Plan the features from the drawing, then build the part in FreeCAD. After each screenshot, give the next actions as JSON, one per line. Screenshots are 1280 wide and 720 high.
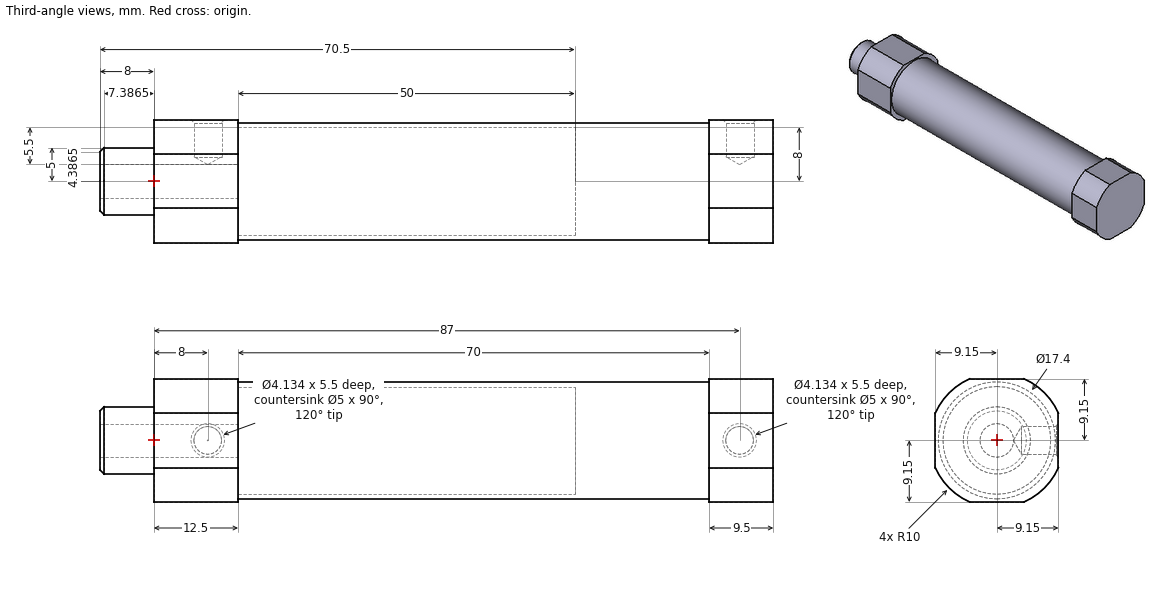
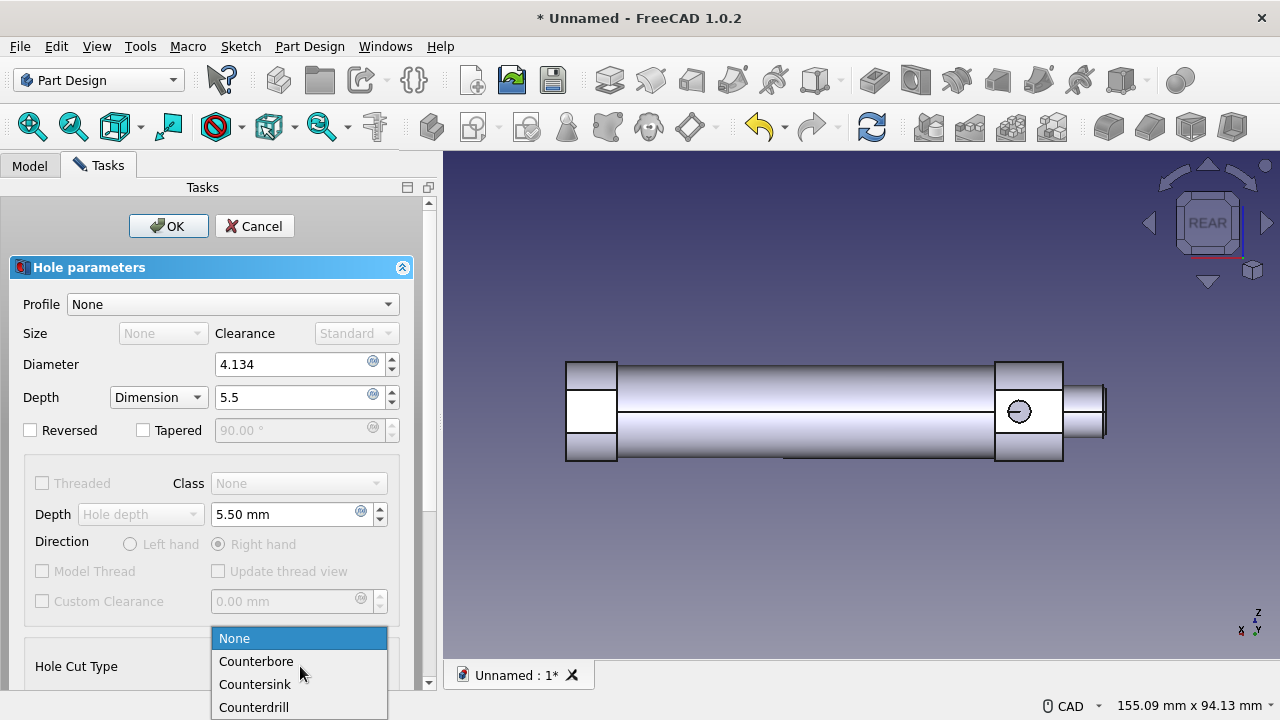
{"action": "left_click", "coordinate": [298, 684]}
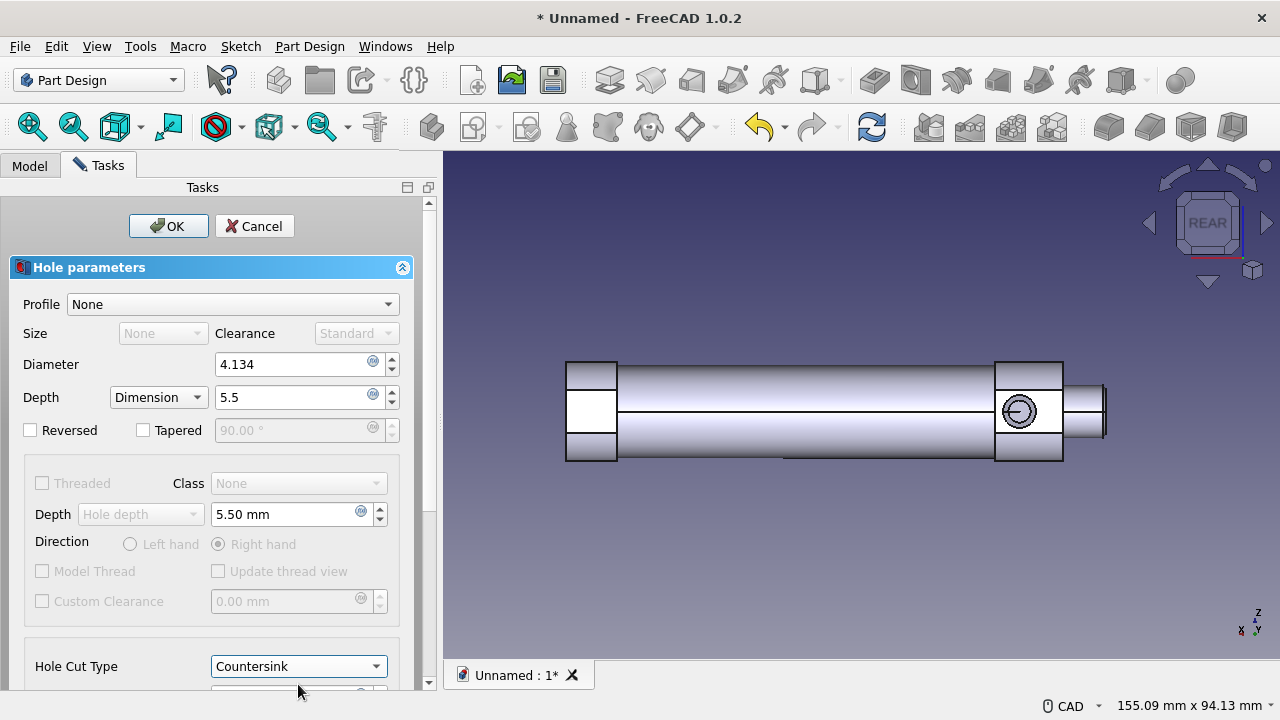
{"action": "scroll", "coordinate": [429, 444], "scroll_direction": "down", "scroll_amount": 2}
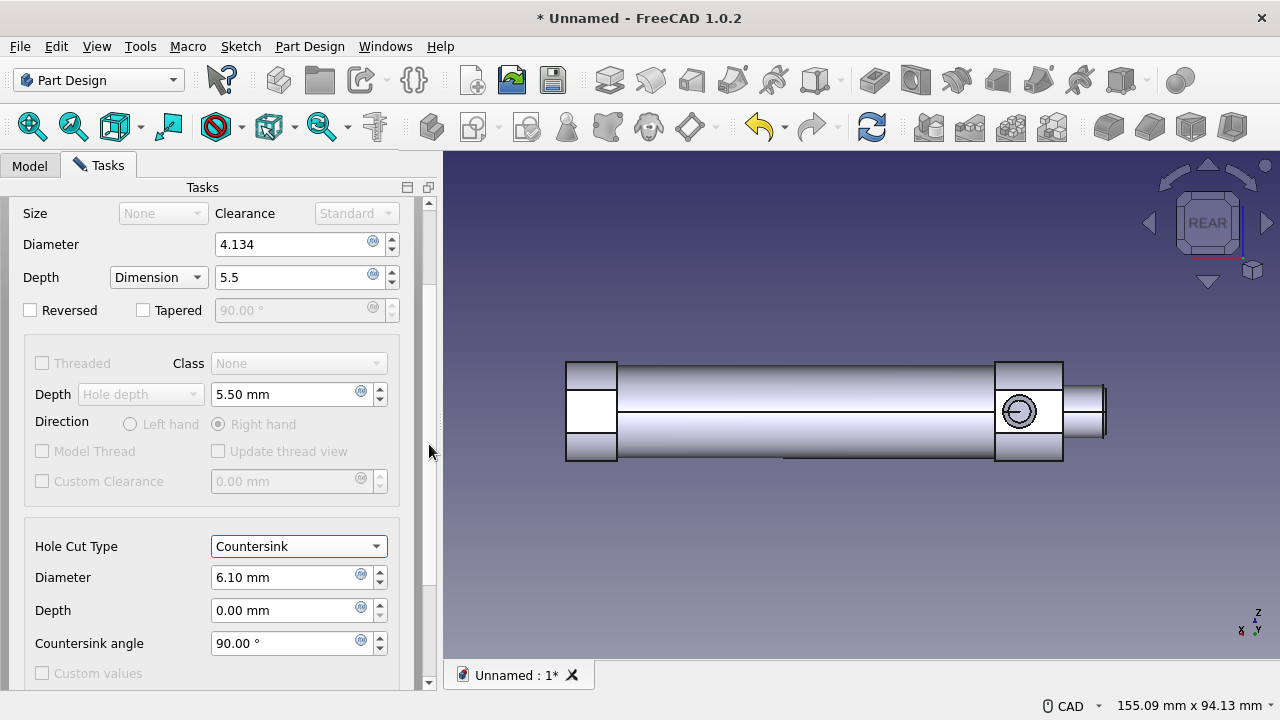
{"action": "triple_click", "coordinate": [292, 578]}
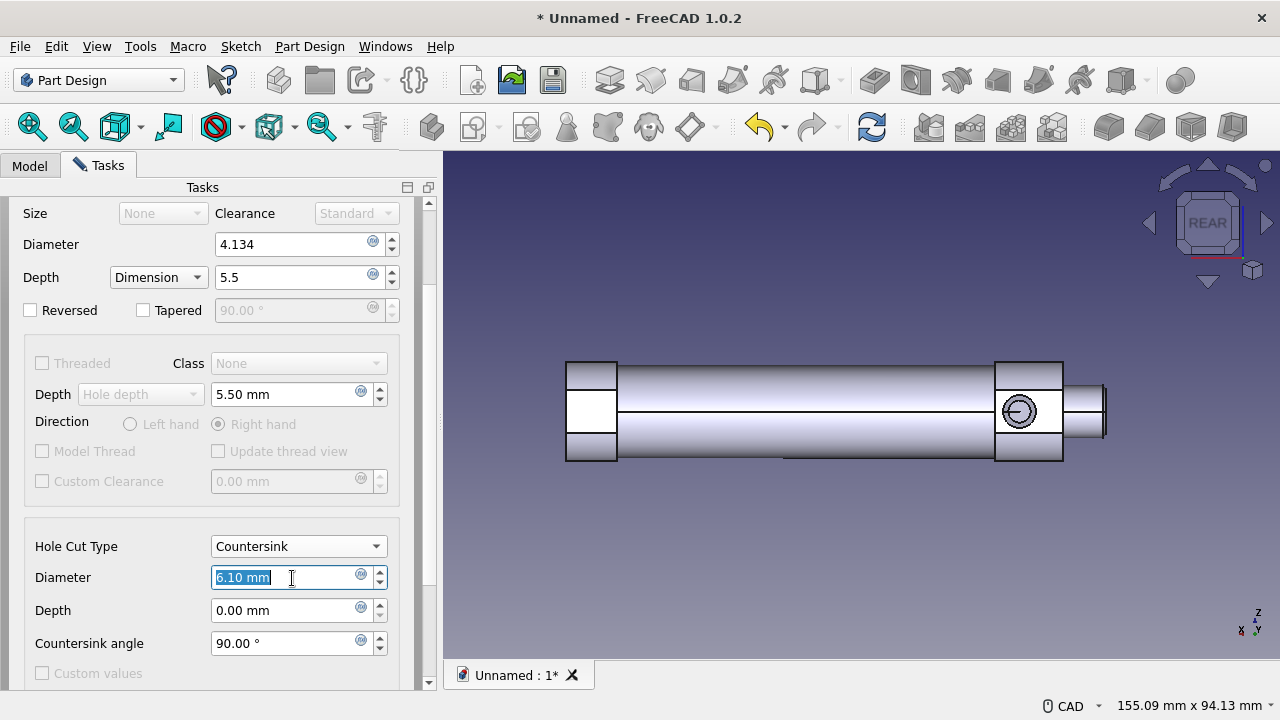
{"action": "type", "text": "5"}
{"action": "key", "text": "Tab"}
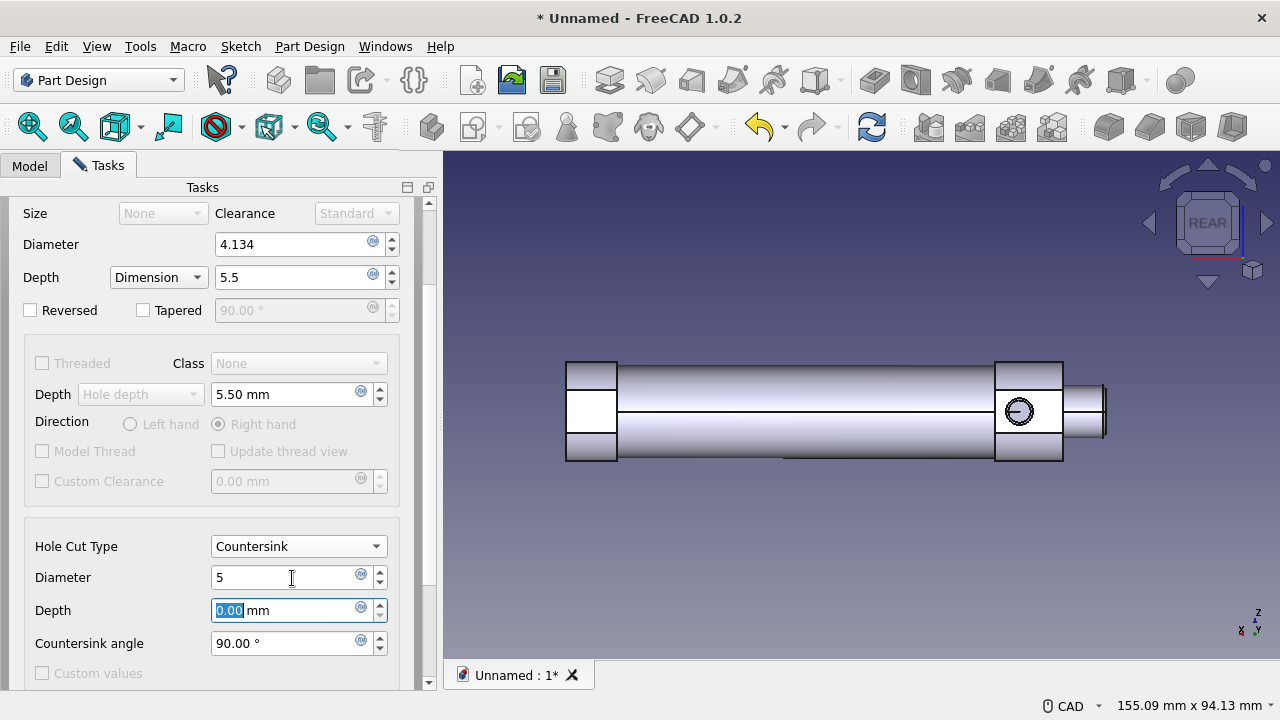
{"action": "scroll", "coordinate": [429, 444], "scroll_direction": "down", "scroll_amount": 3}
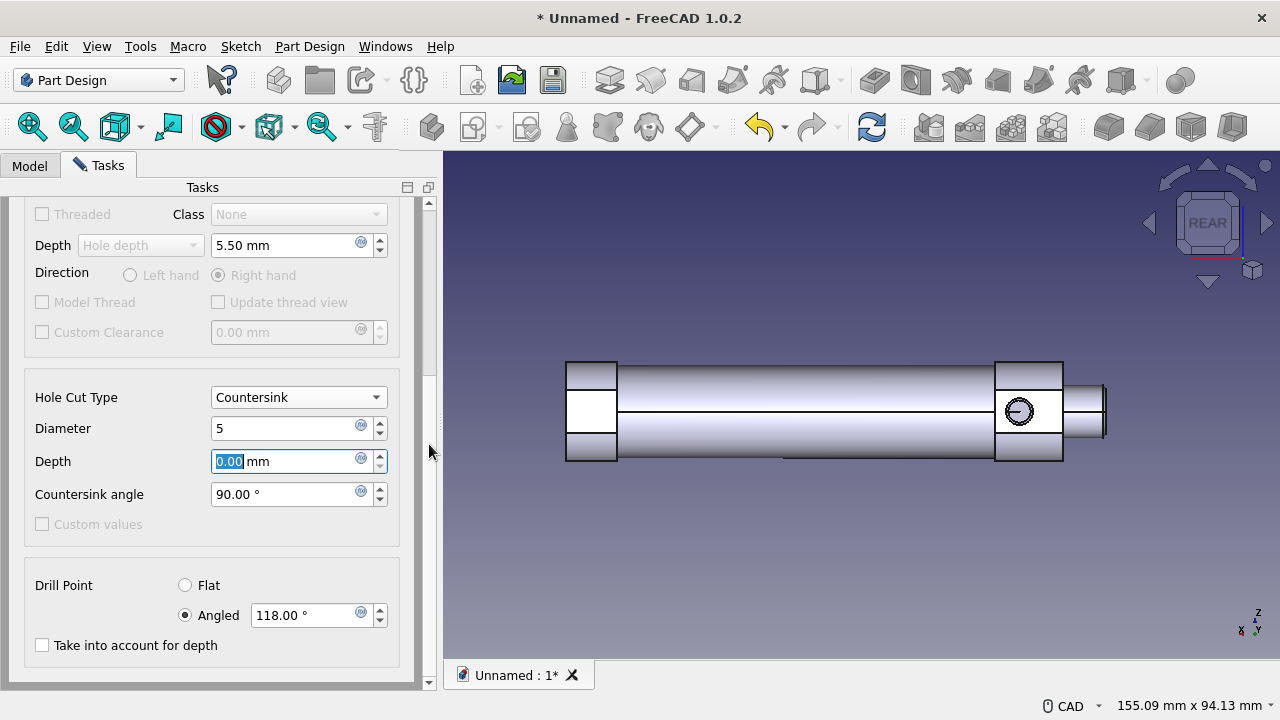
{"action": "triple_click", "coordinate": [312, 616]}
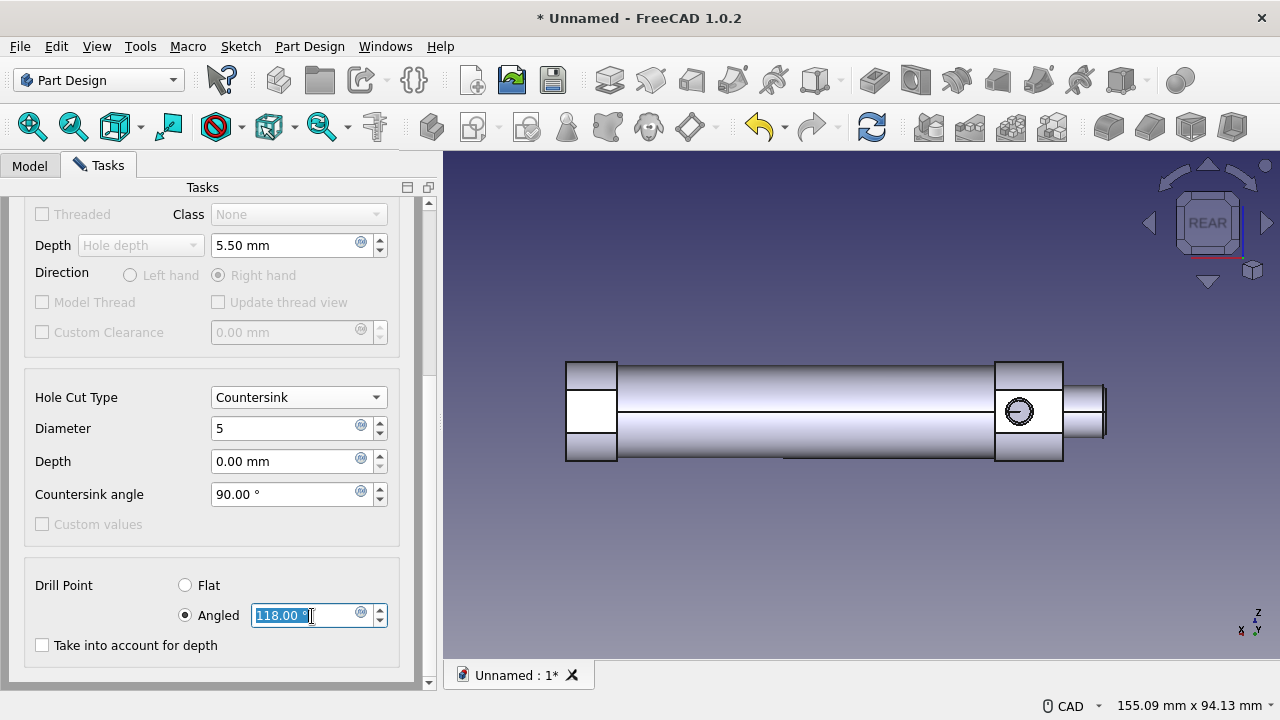
{"action": "type", "text": "120"}
{"action": "key", "text": "Tab"}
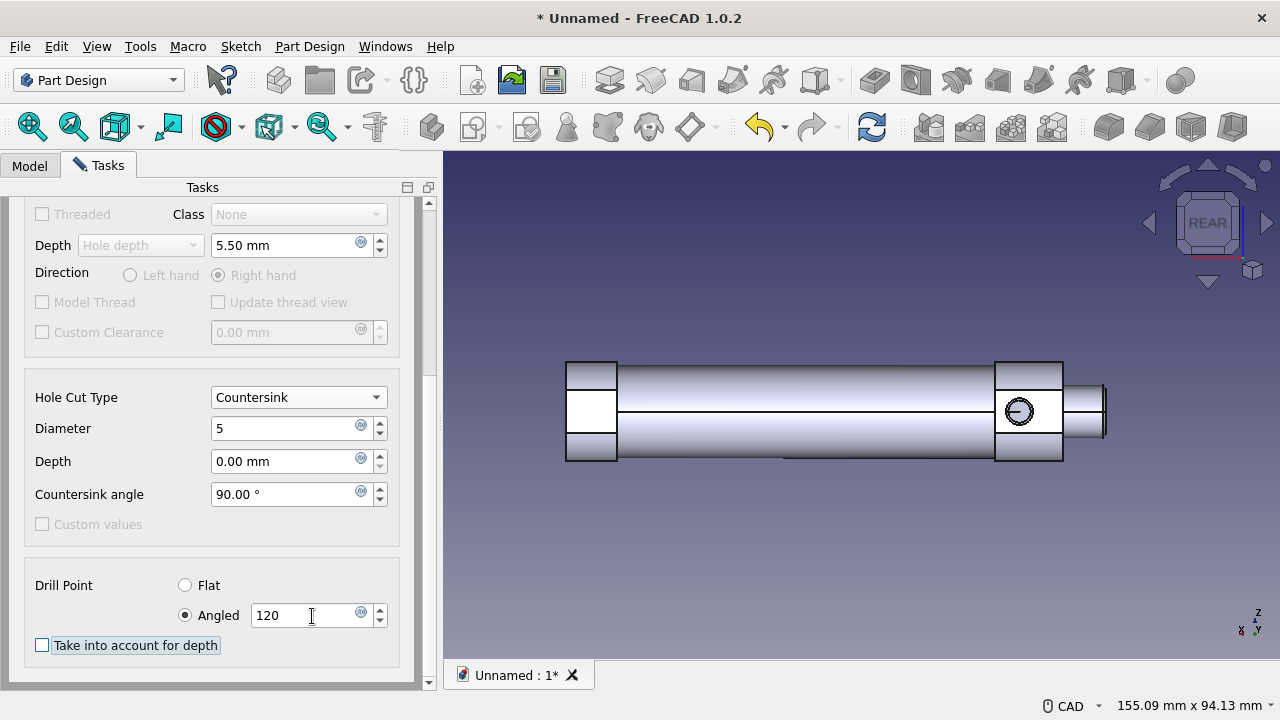
{"action": "scroll", "coordinate": [429, 444], "scroll_direction": "up", "scroll_amount": 6}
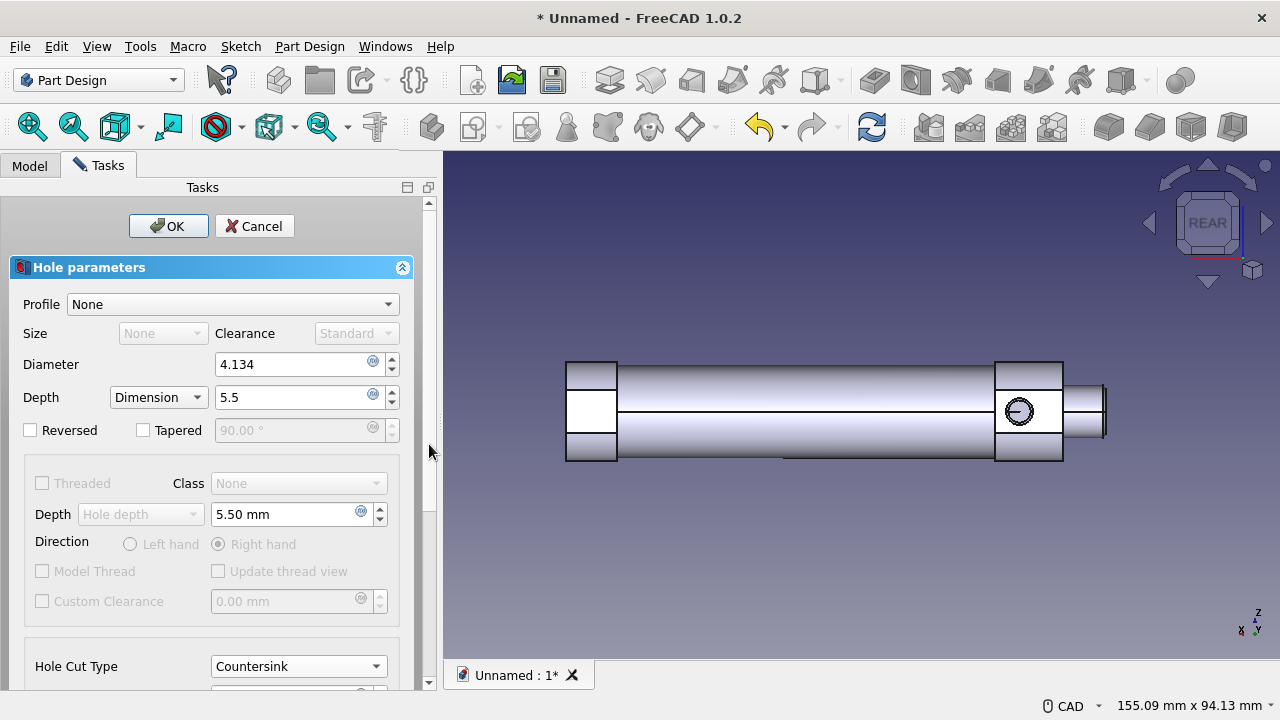
{"action": "left_click", "coordinate": [169, 226]}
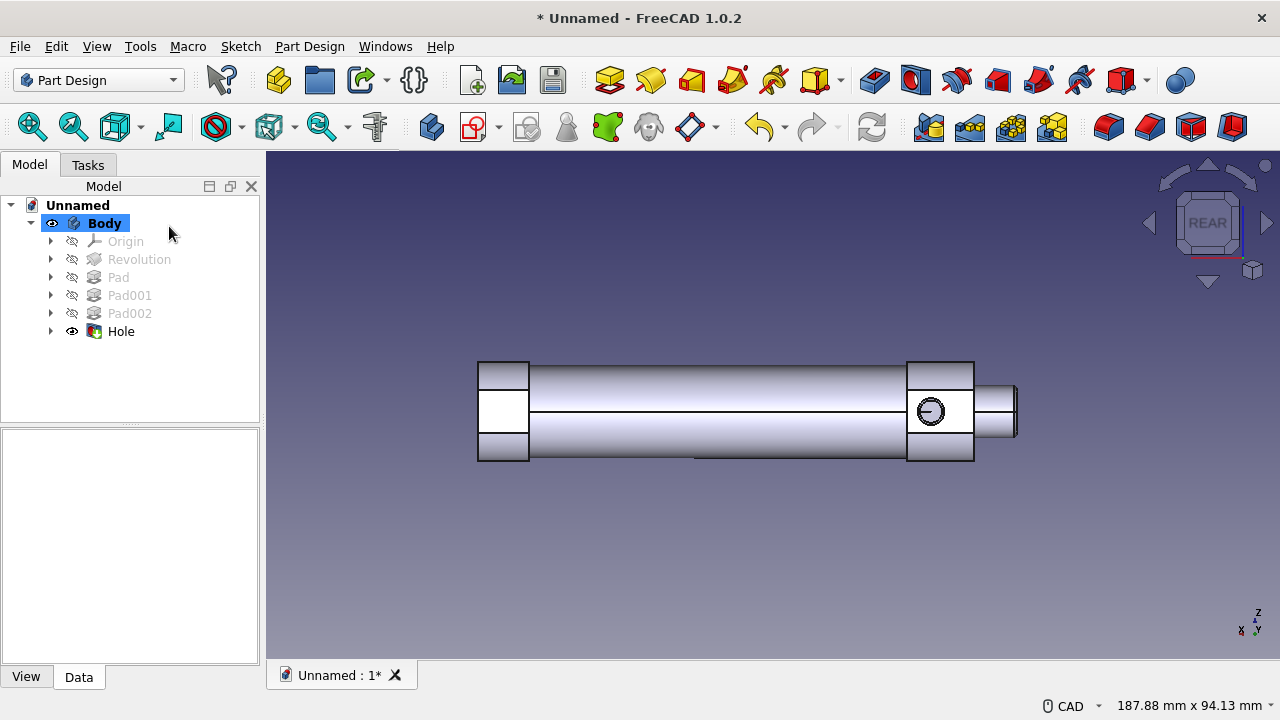
{"action": "left_click", "coordinate": [960, 404]}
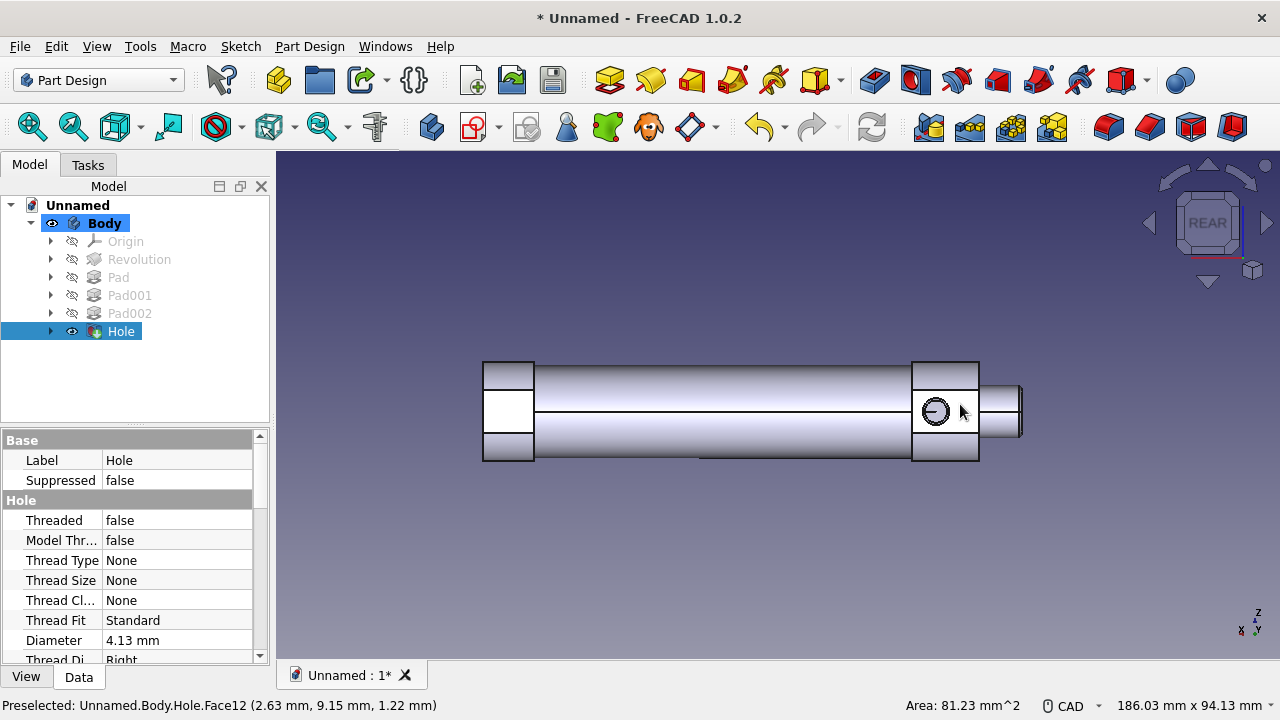
{"action": "left_click", "coordinate": [472, 128]}